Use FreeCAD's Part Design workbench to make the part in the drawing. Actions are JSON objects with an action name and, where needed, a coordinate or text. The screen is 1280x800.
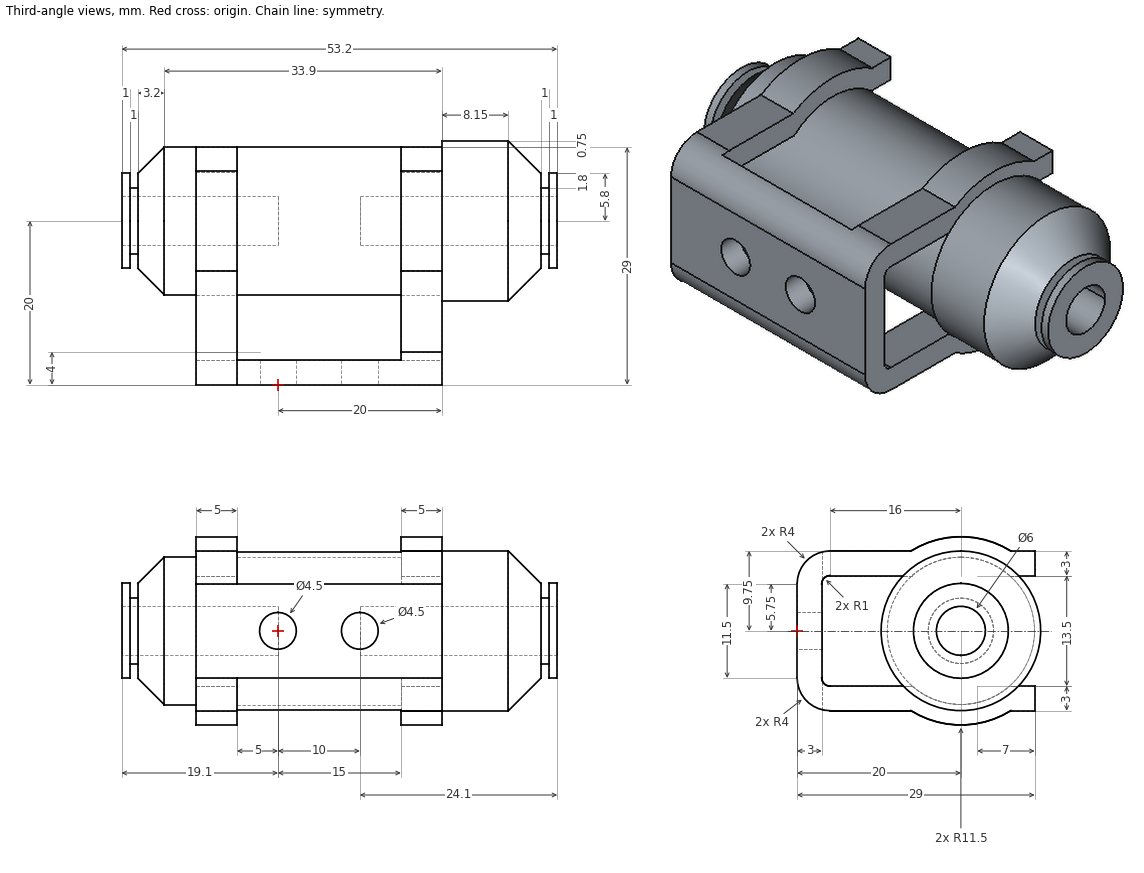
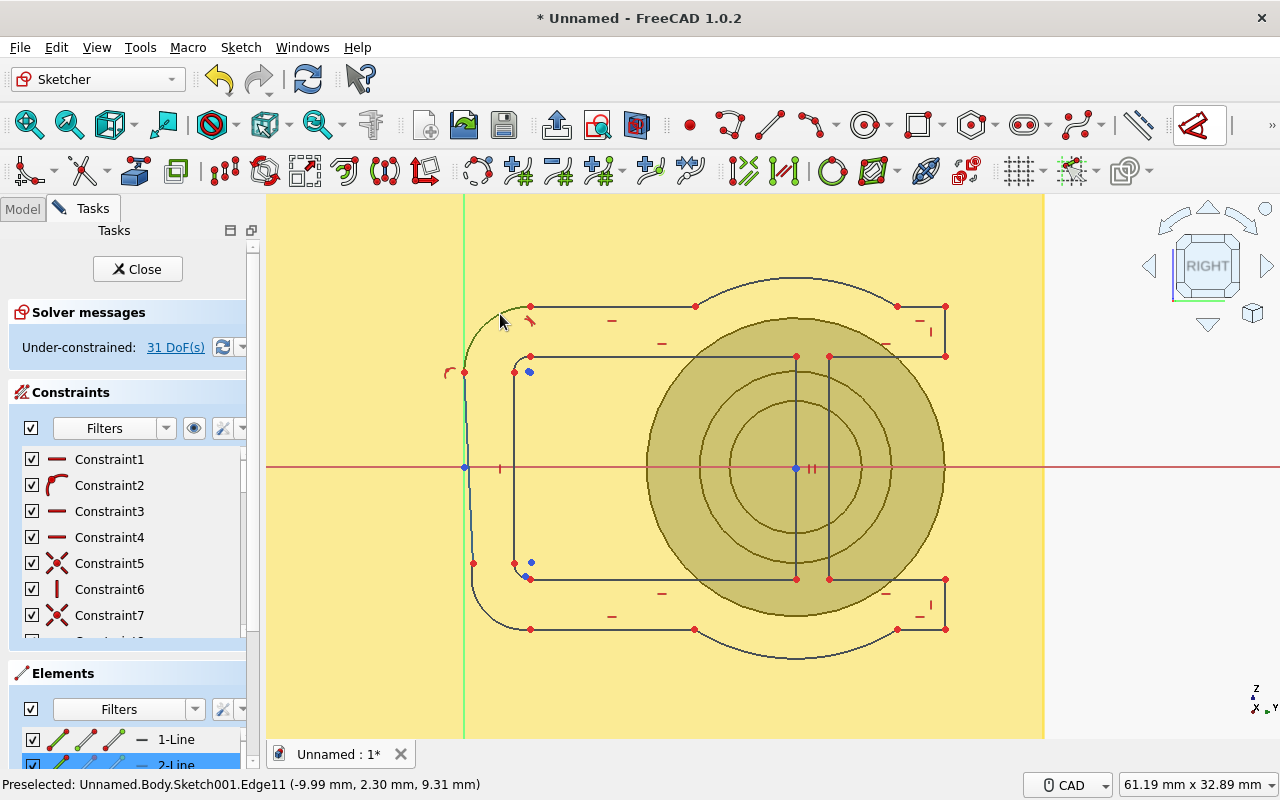
{"action": "key", "text": "t"}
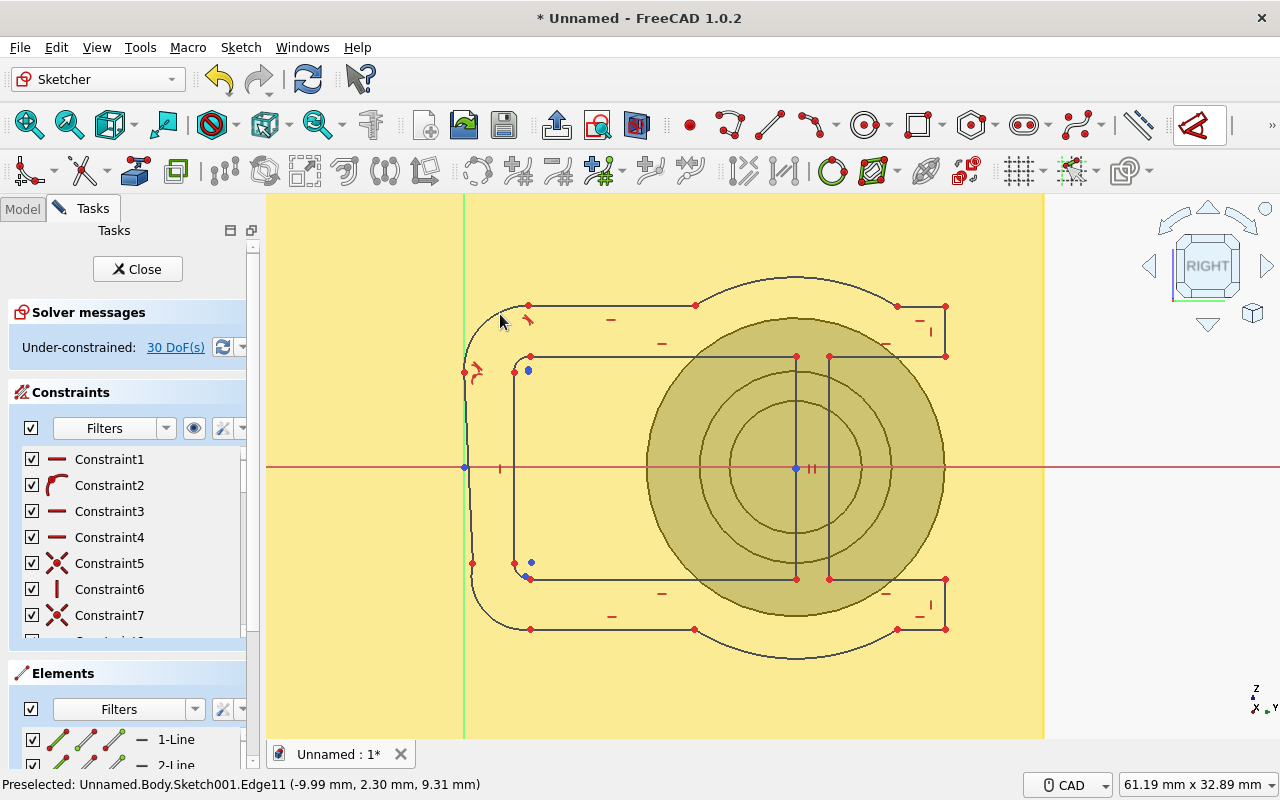
{"action": "left_click", "coordinate": [467, 430]}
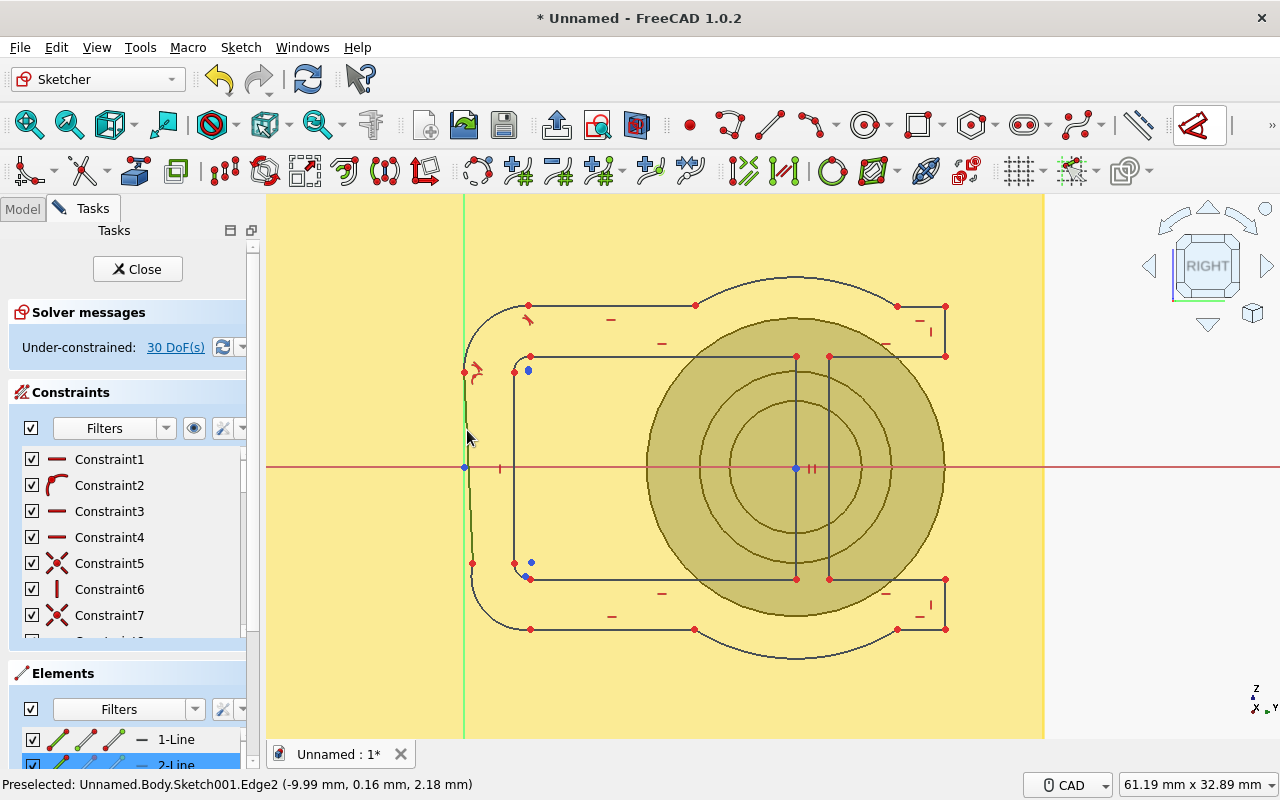
{"action": "scroll", "coordinate": [474, 594], "scroll_direction": "up", "scroll_amount": 2}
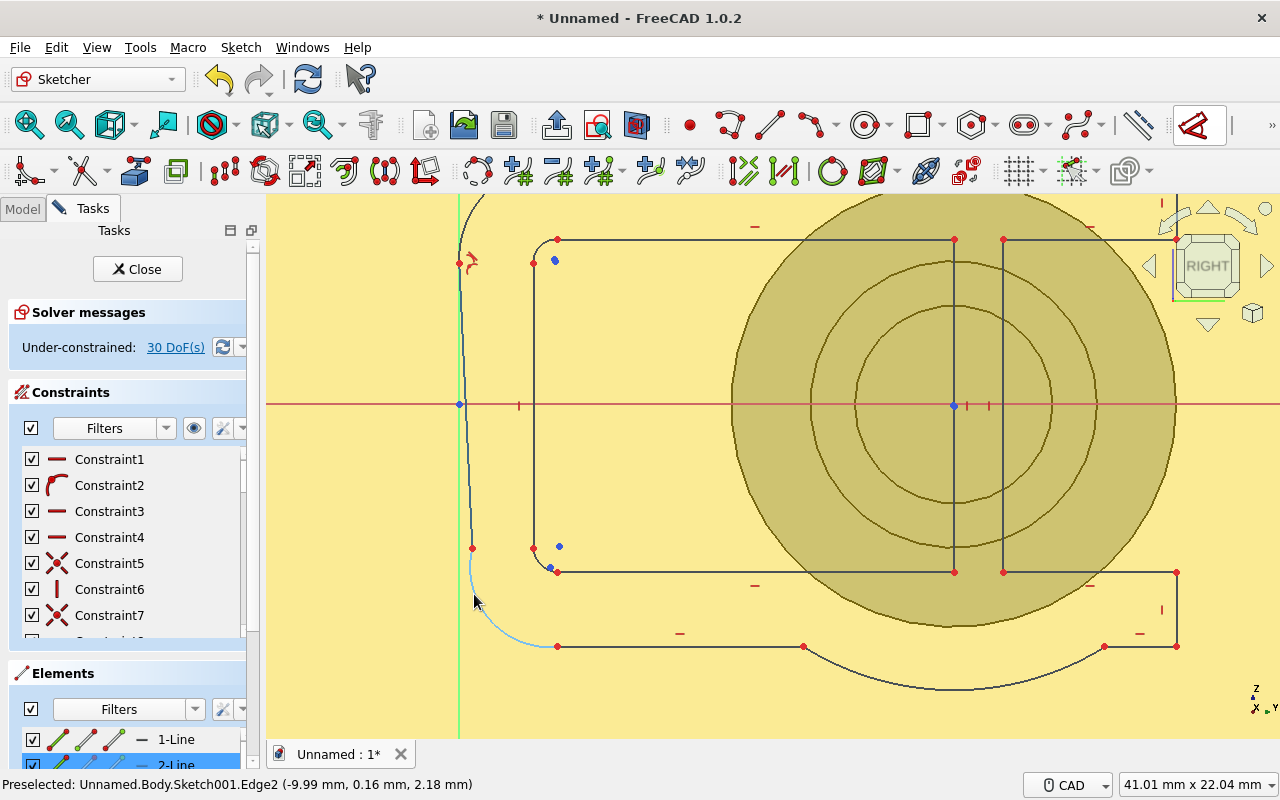
{"action": "left_click", "coordinate": [475, 593]}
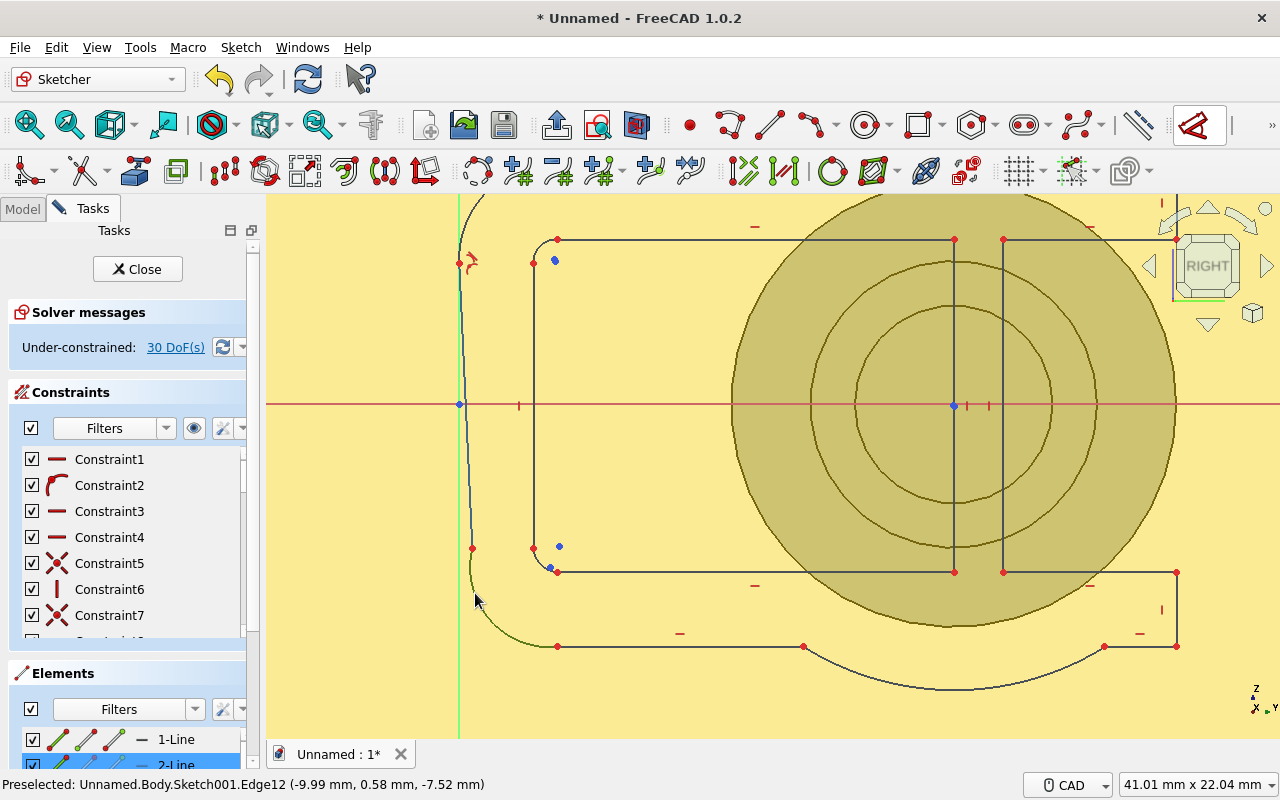
{"action": "key", "text": "t"}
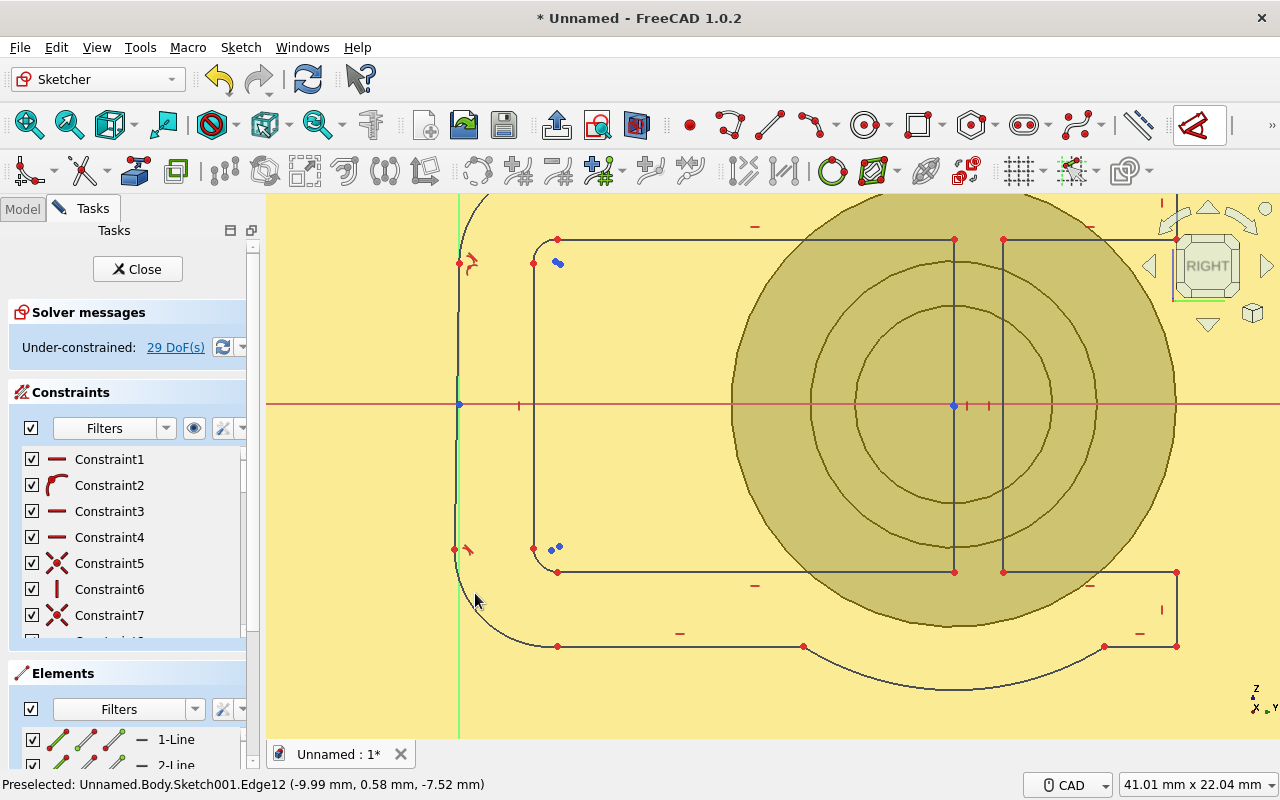
{"action": "left_click", "coordinate": [631, 647]}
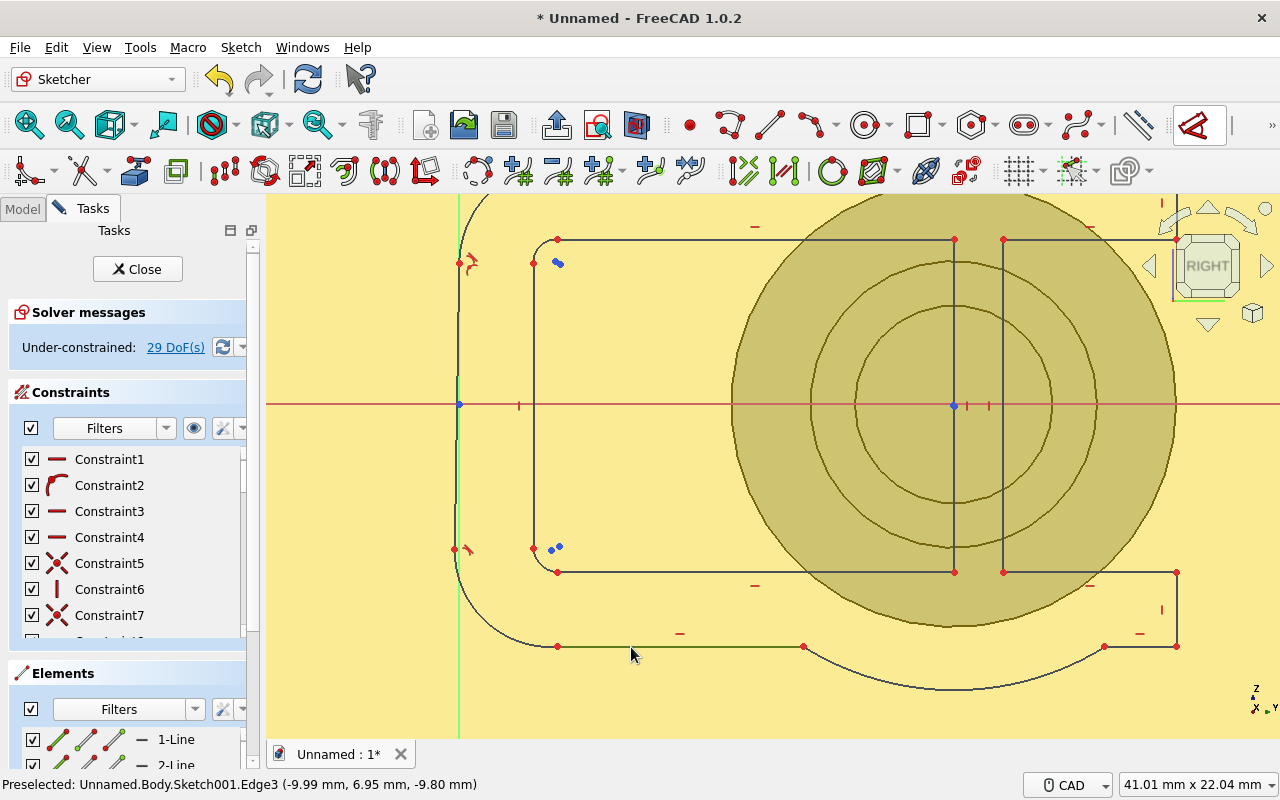
{"action": "left_click", "coordinate": [511, 638]}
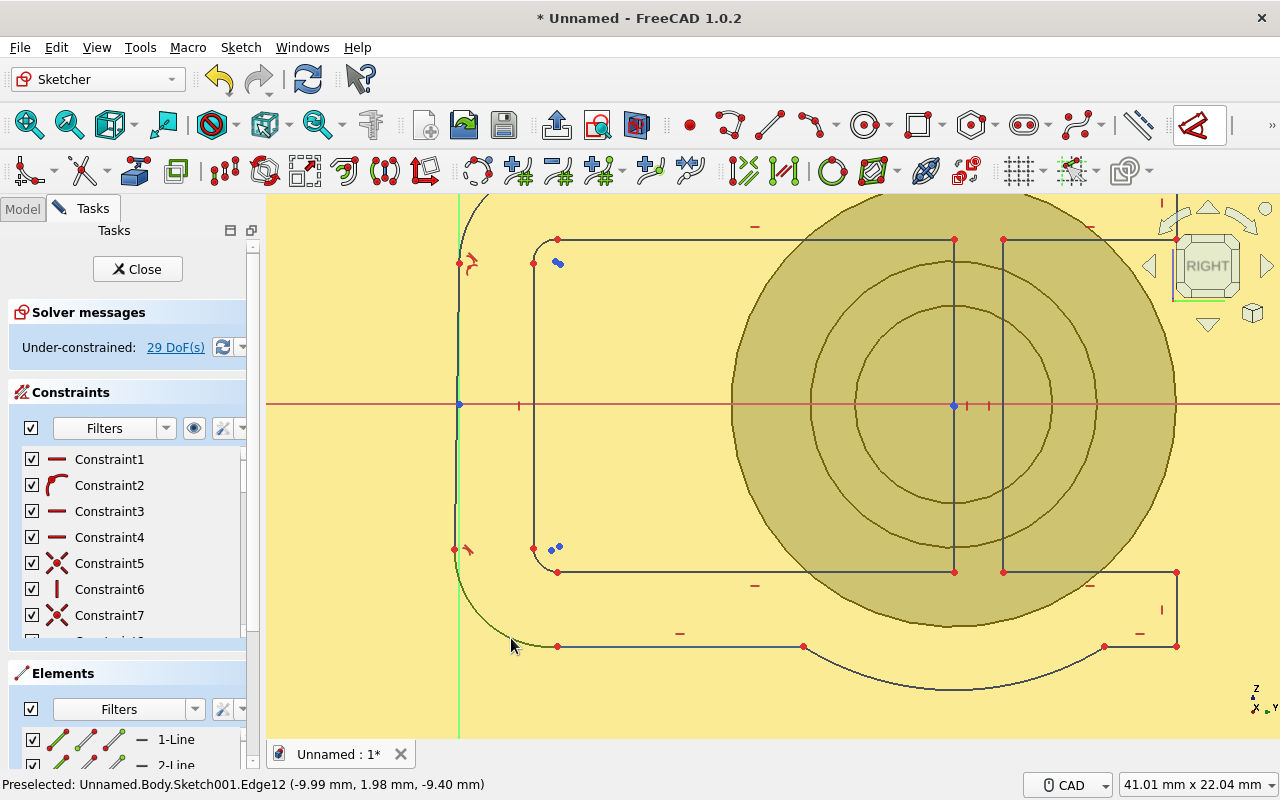
{"action": "key", "text": "t"}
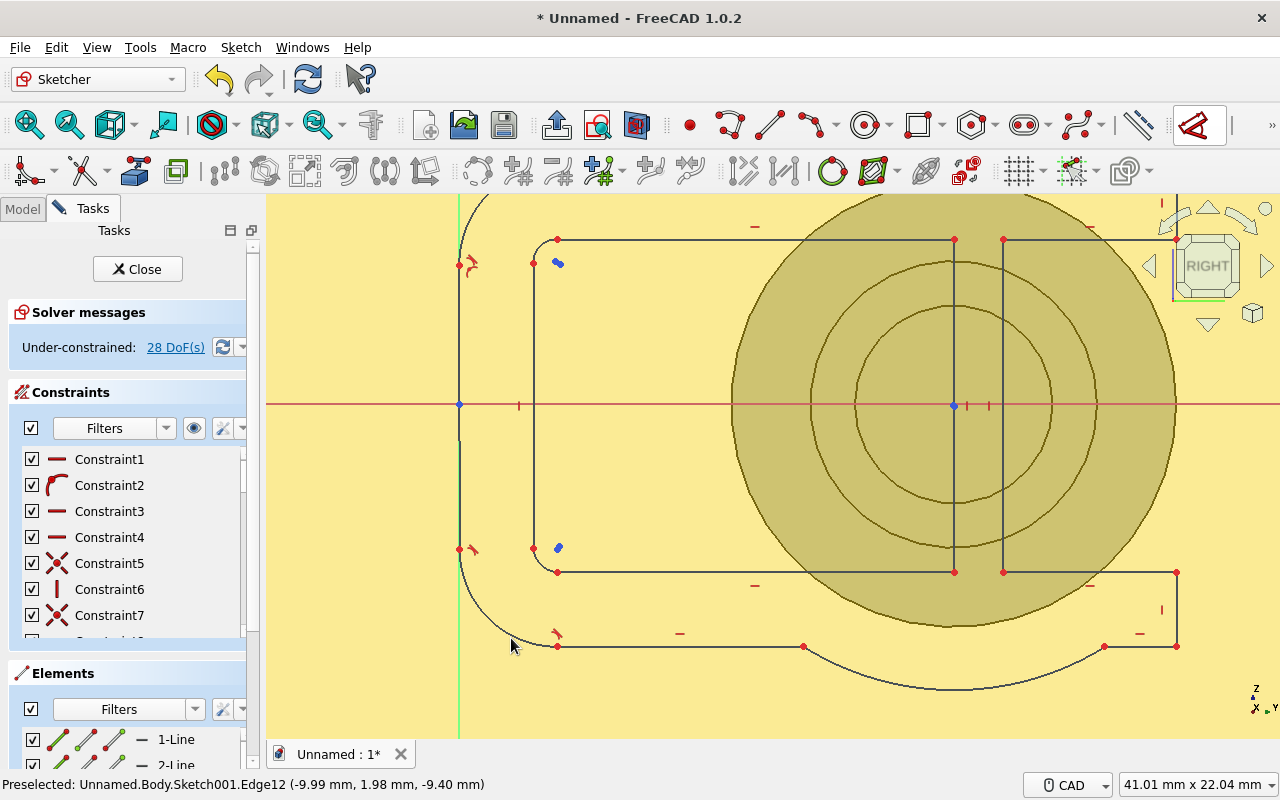
{"action": "left_click", "coordinate": [534, 463]}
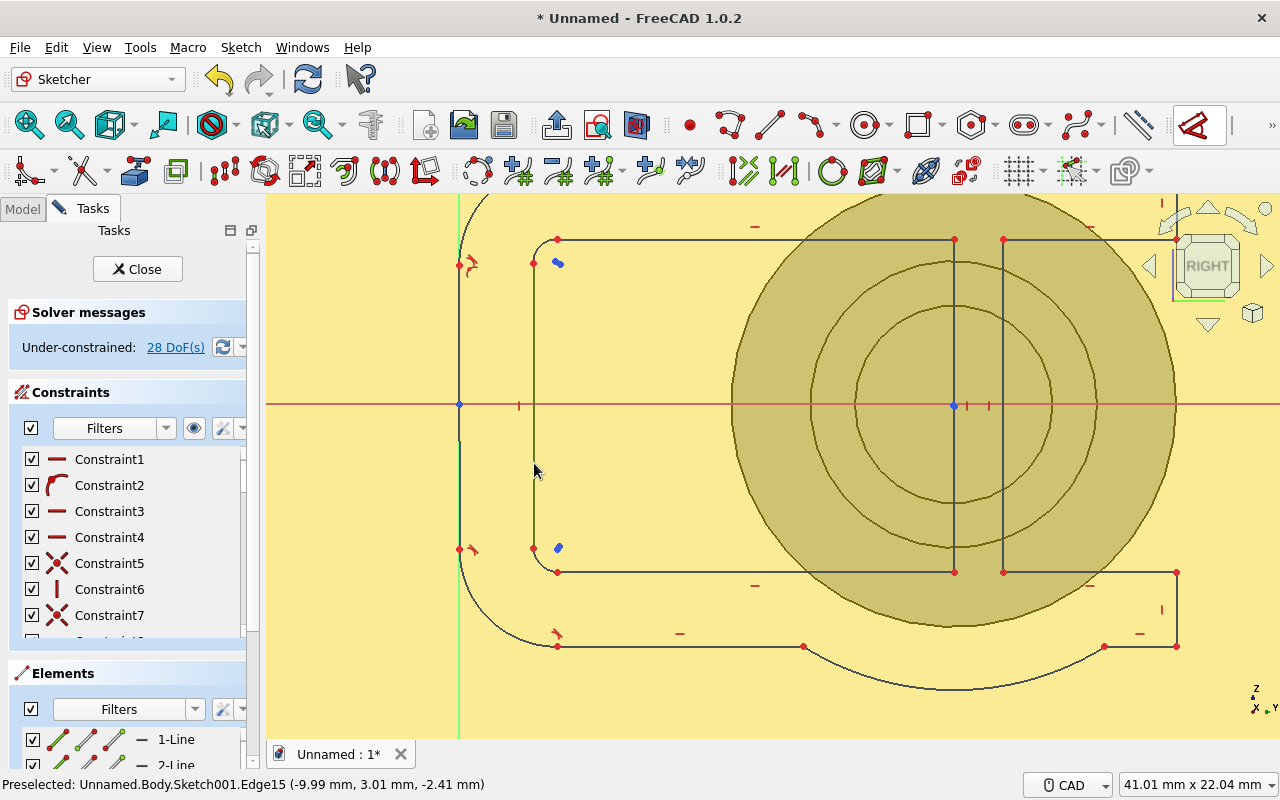
{"action": "left_click", "coordinate": [546, 242]}